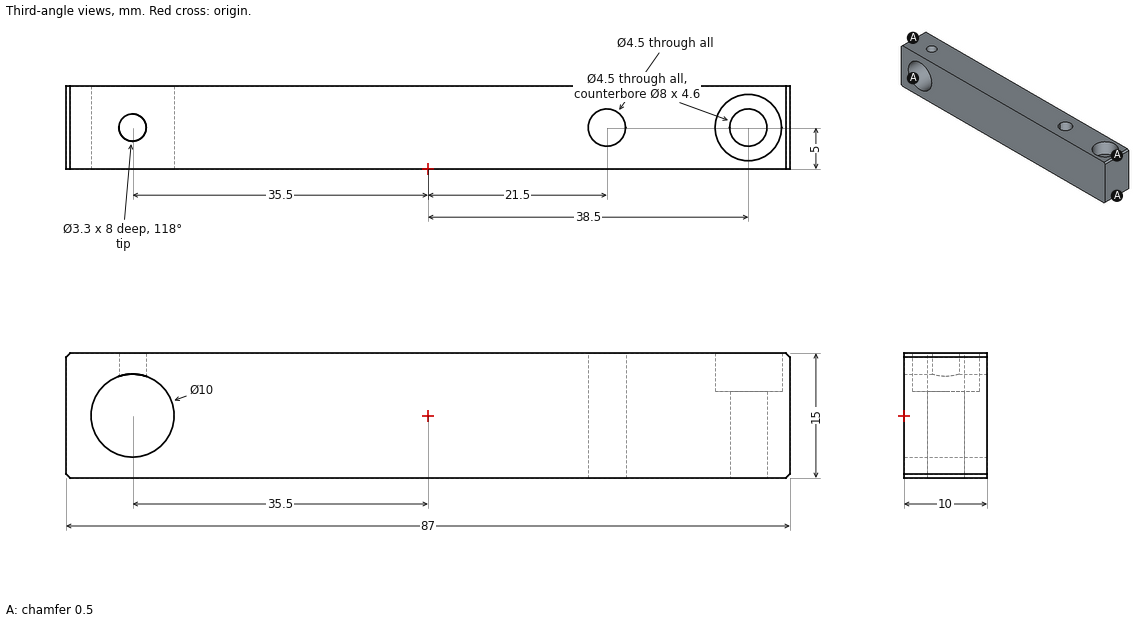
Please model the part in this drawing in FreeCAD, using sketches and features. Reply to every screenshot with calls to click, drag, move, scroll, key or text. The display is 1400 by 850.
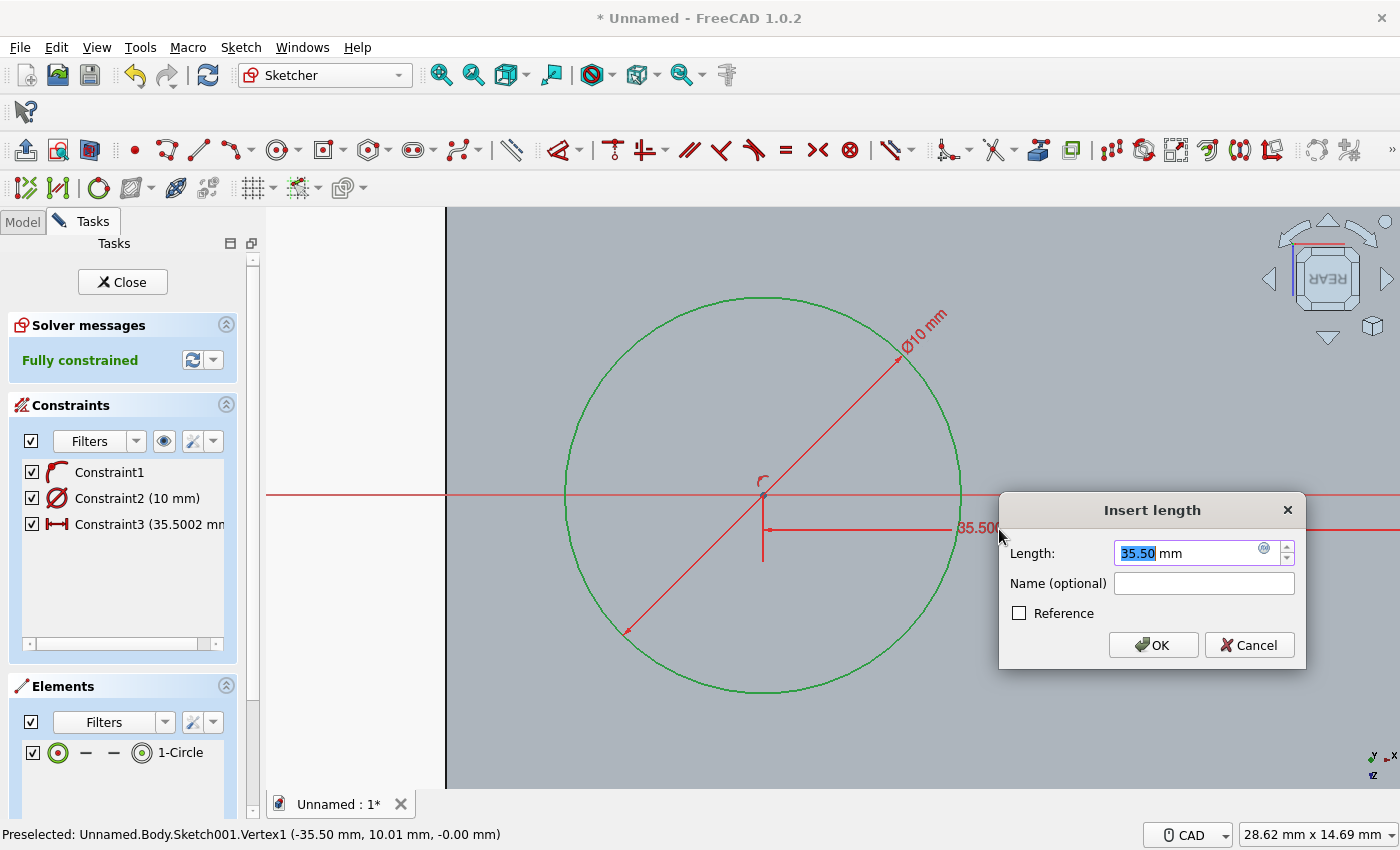
text(35.5)
key(Return)
key(Escape)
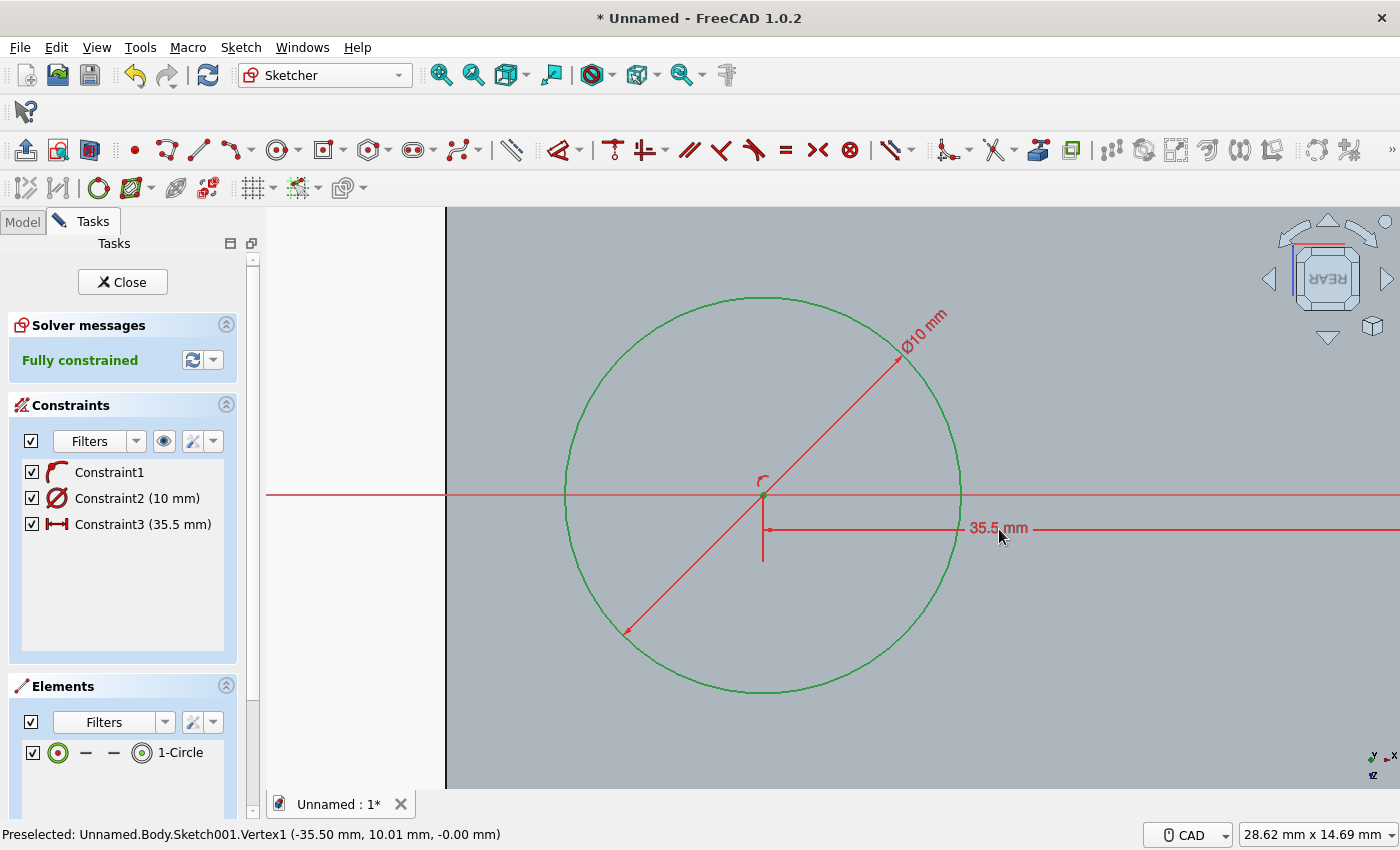
click(123, 282)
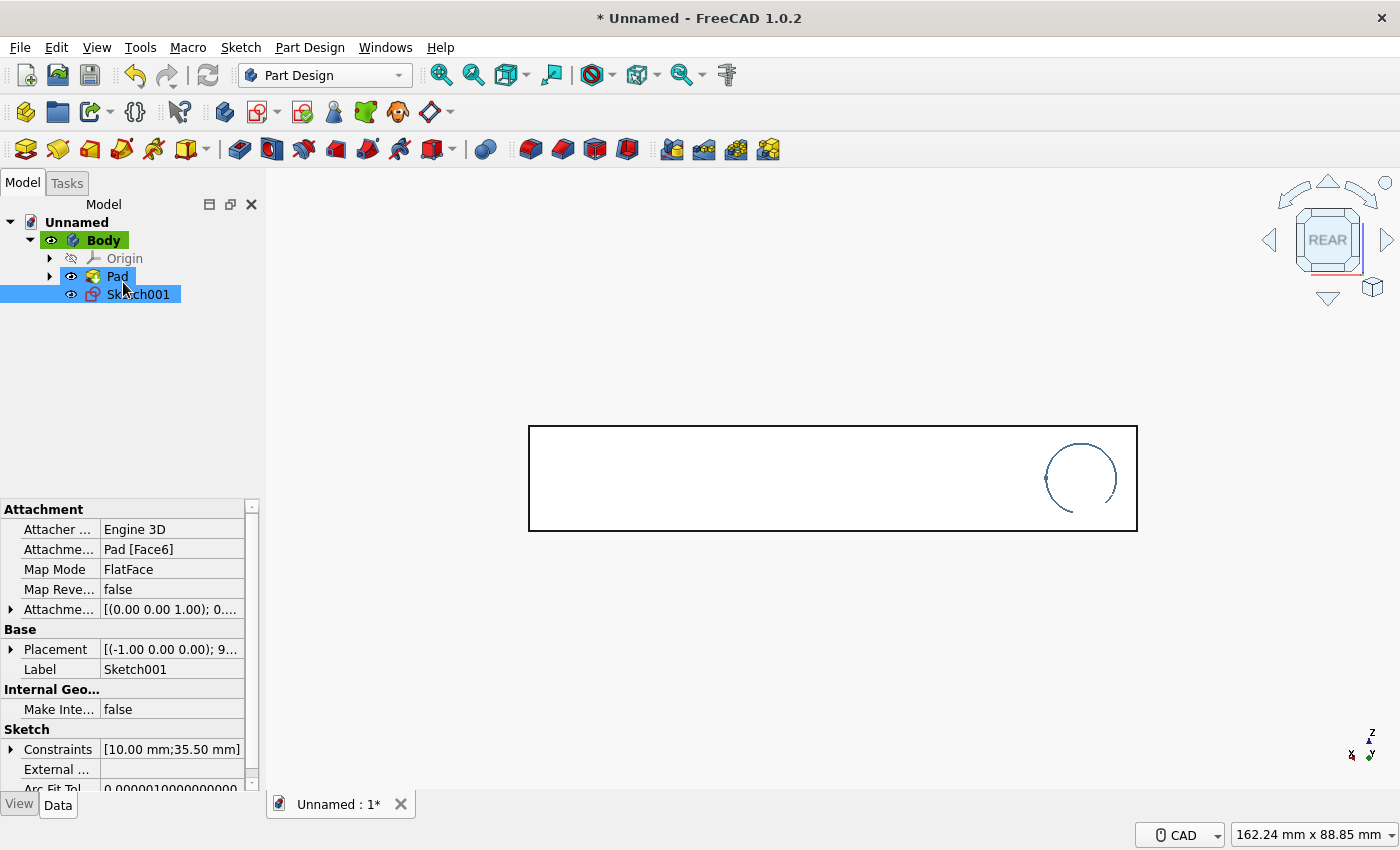
click(240, 150)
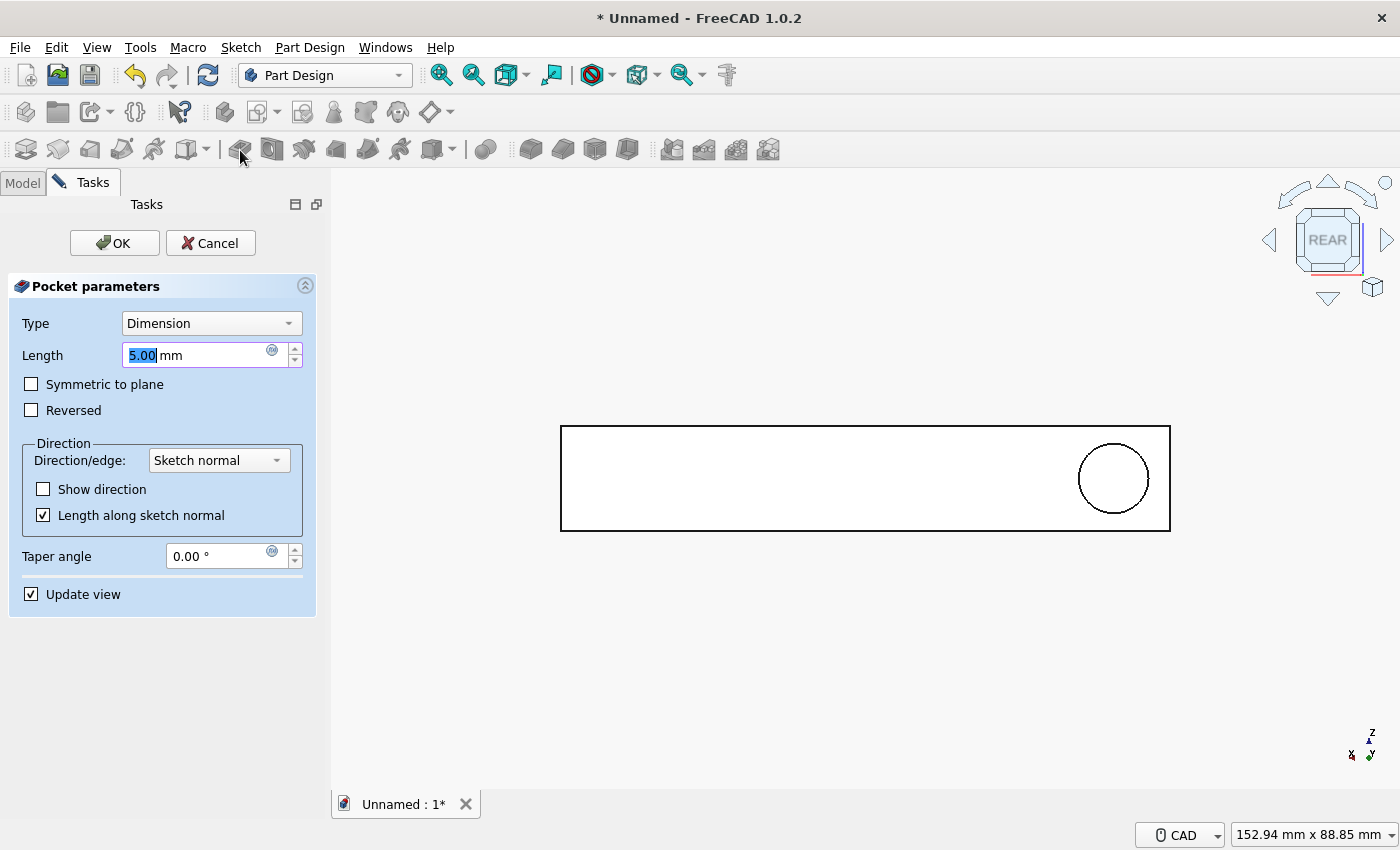
click(212, 324)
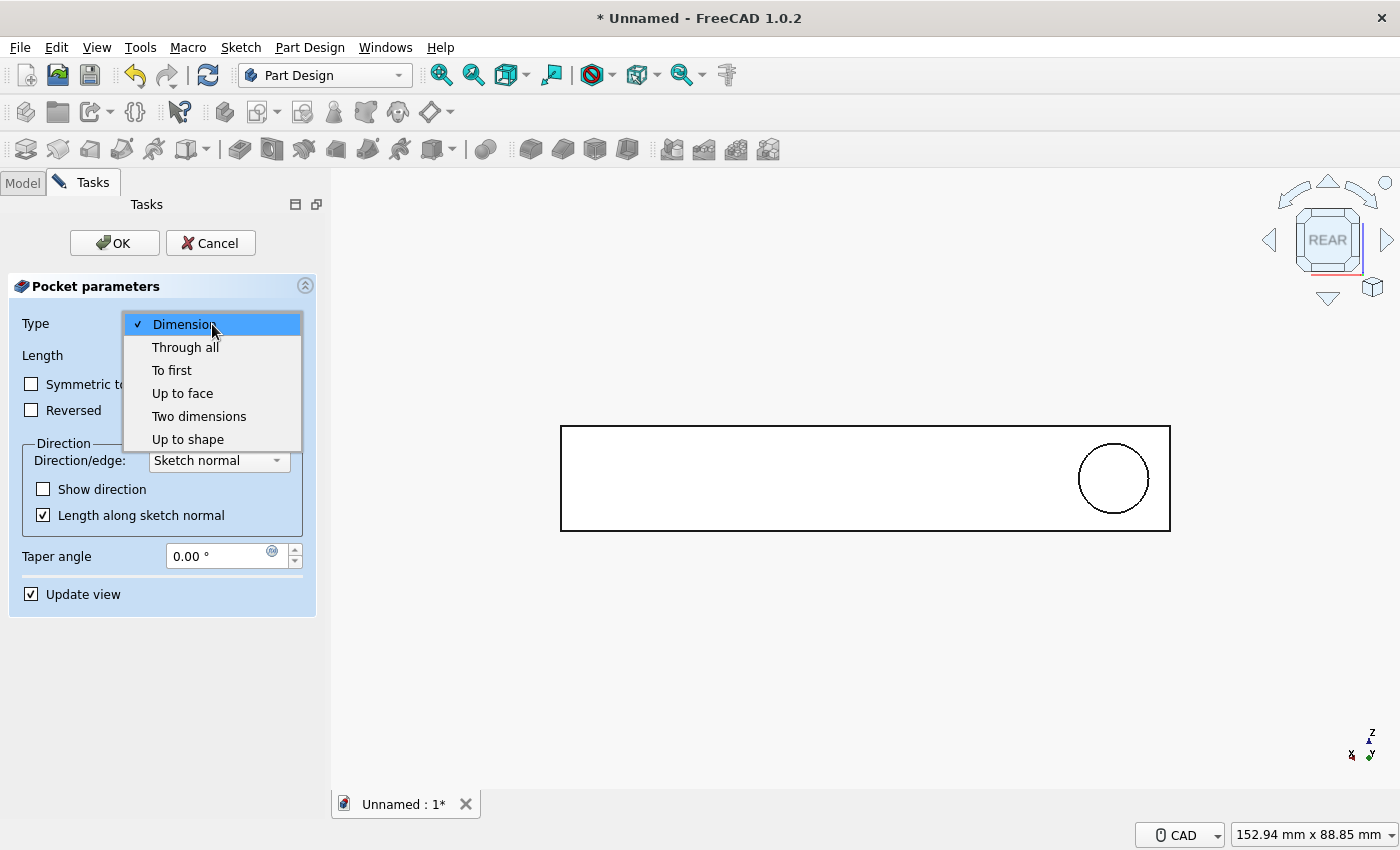
click(212, 348)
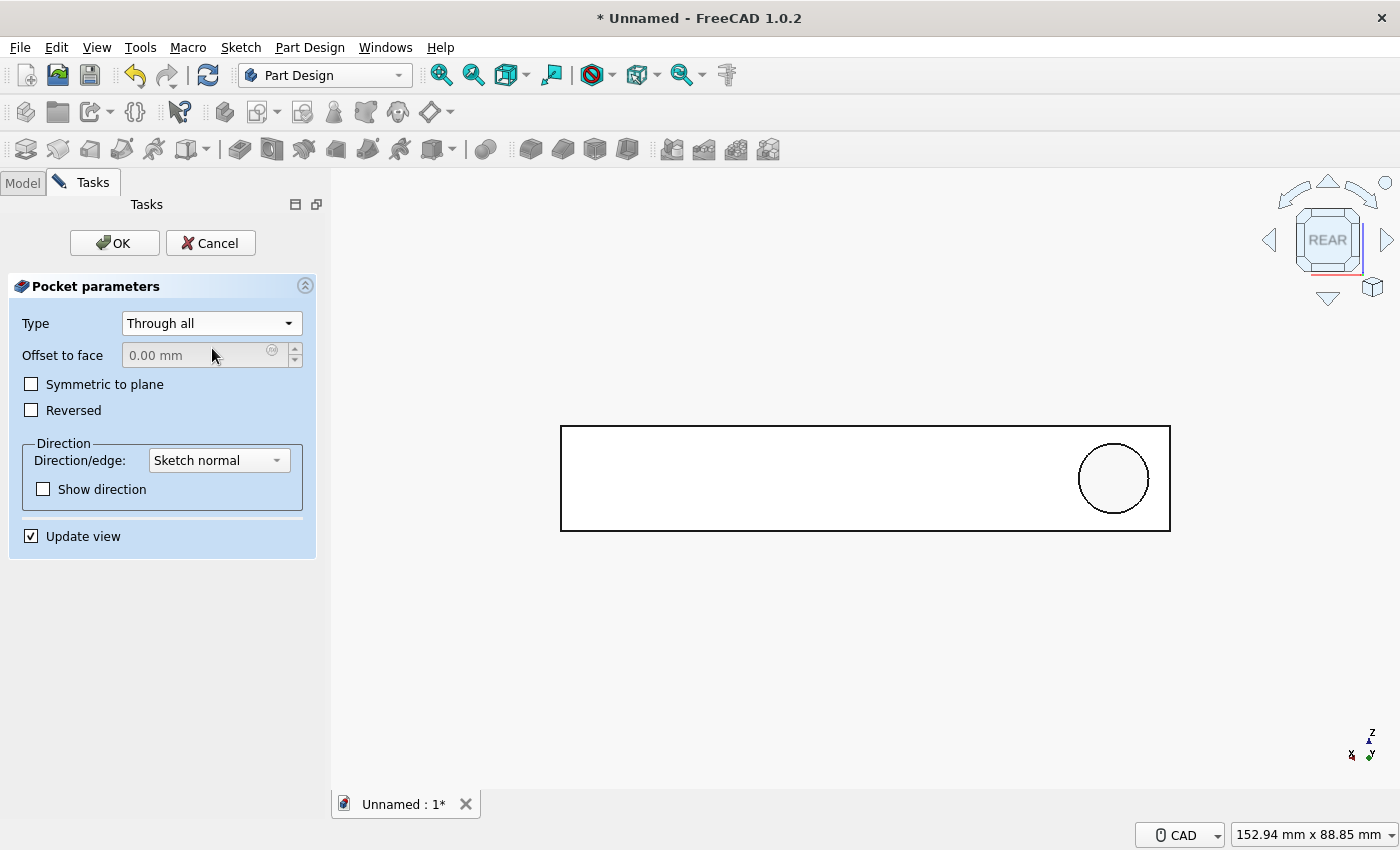
click(115, 243)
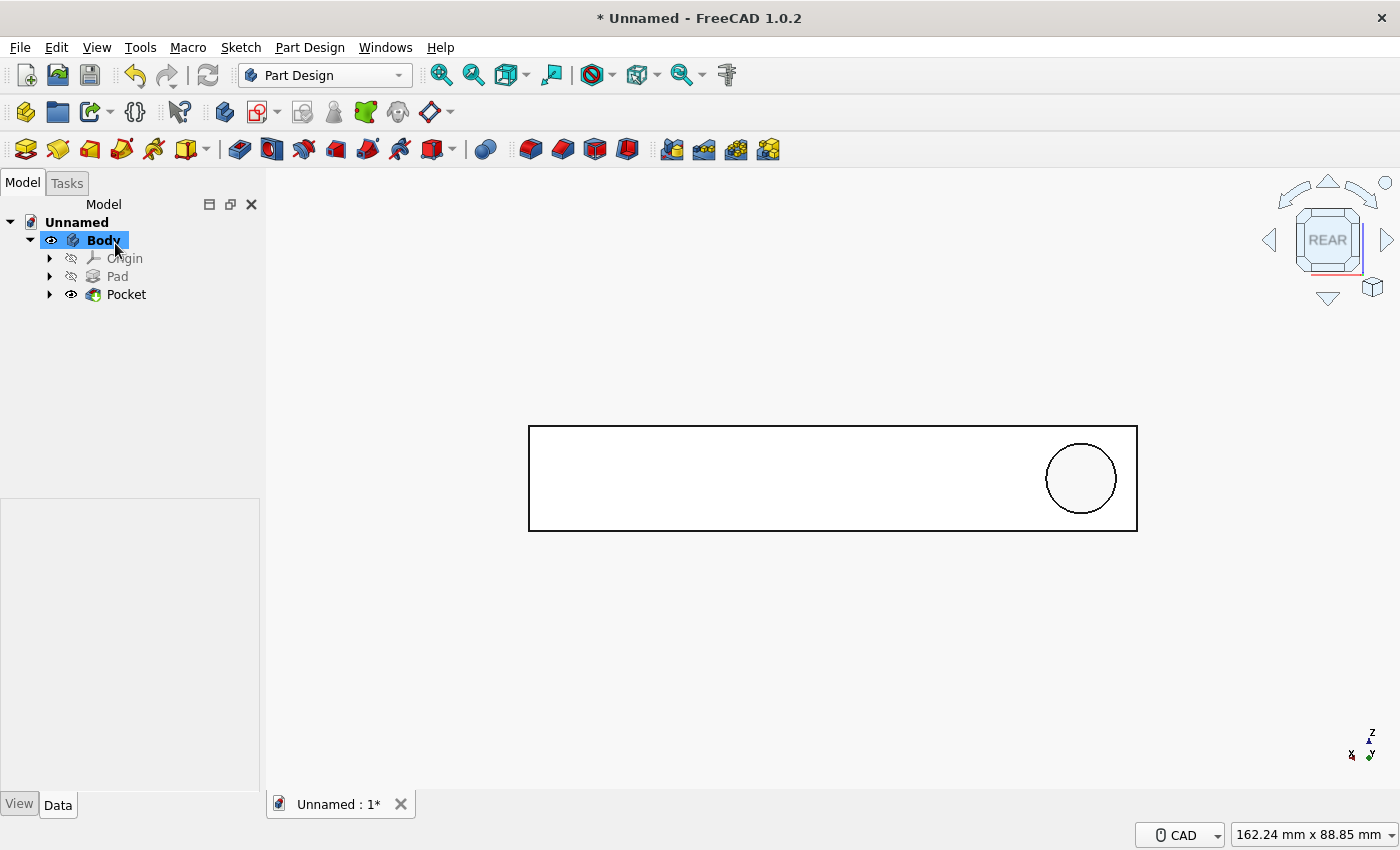
key(5)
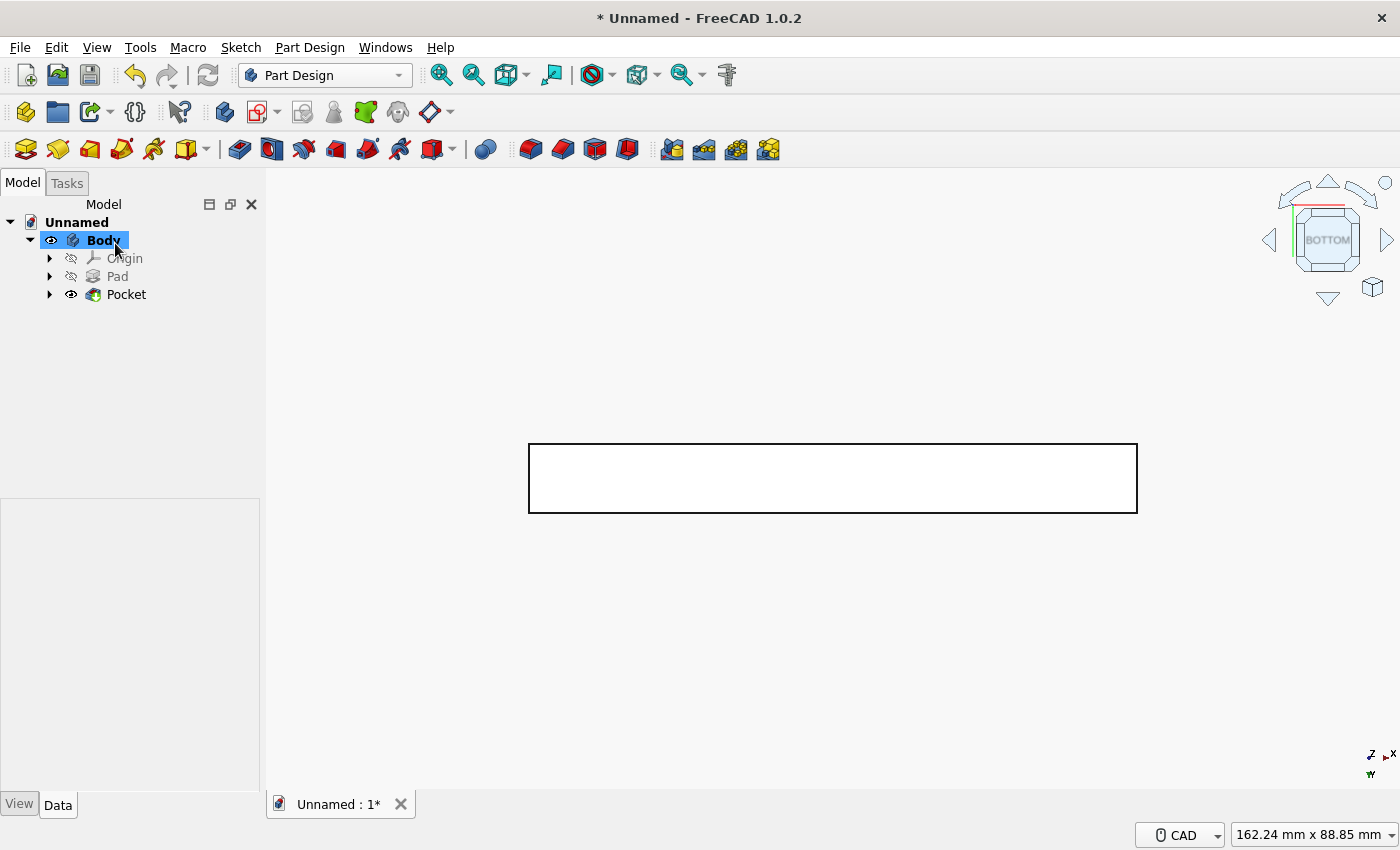
click(1094, 478)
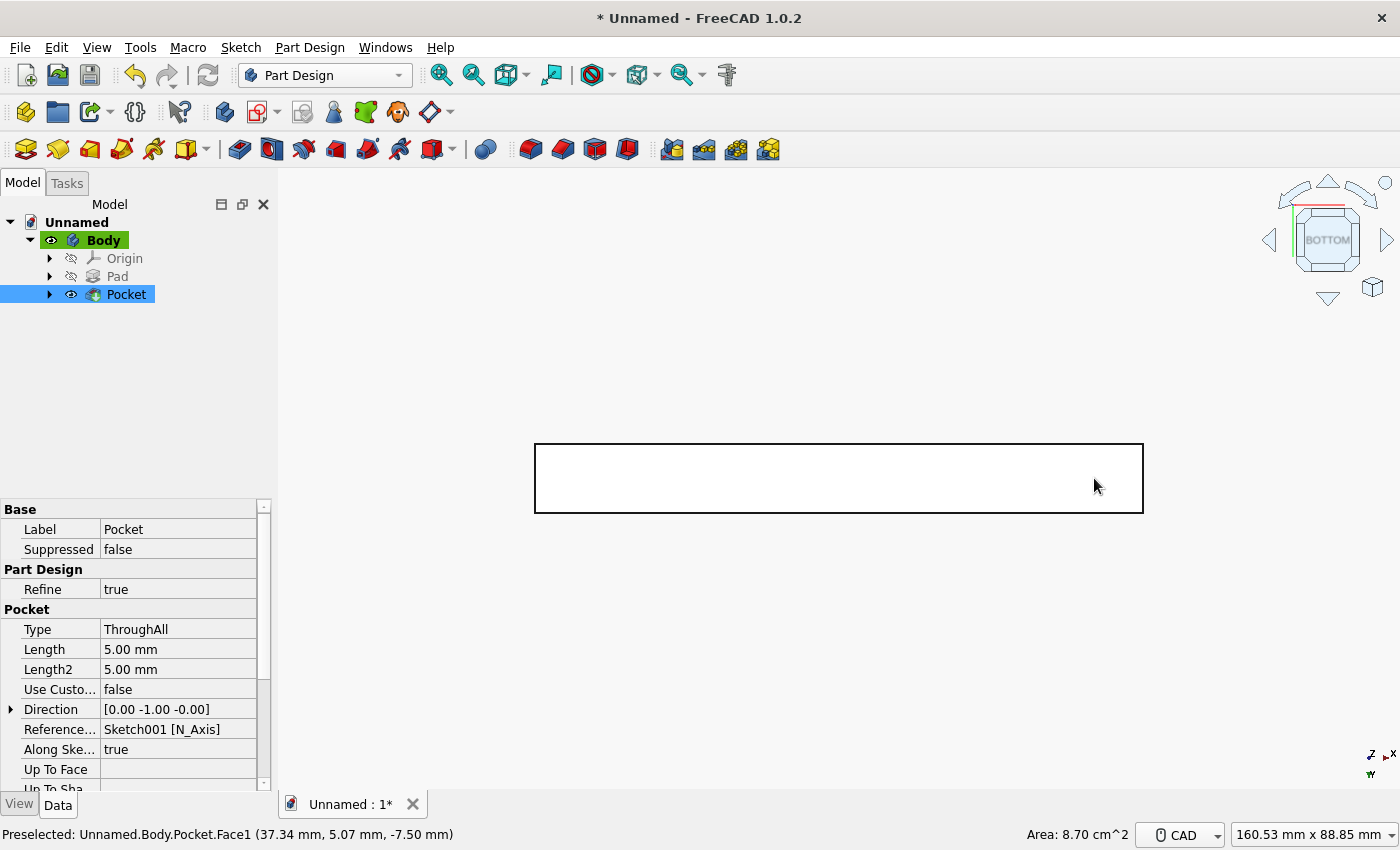
click(258, 112)